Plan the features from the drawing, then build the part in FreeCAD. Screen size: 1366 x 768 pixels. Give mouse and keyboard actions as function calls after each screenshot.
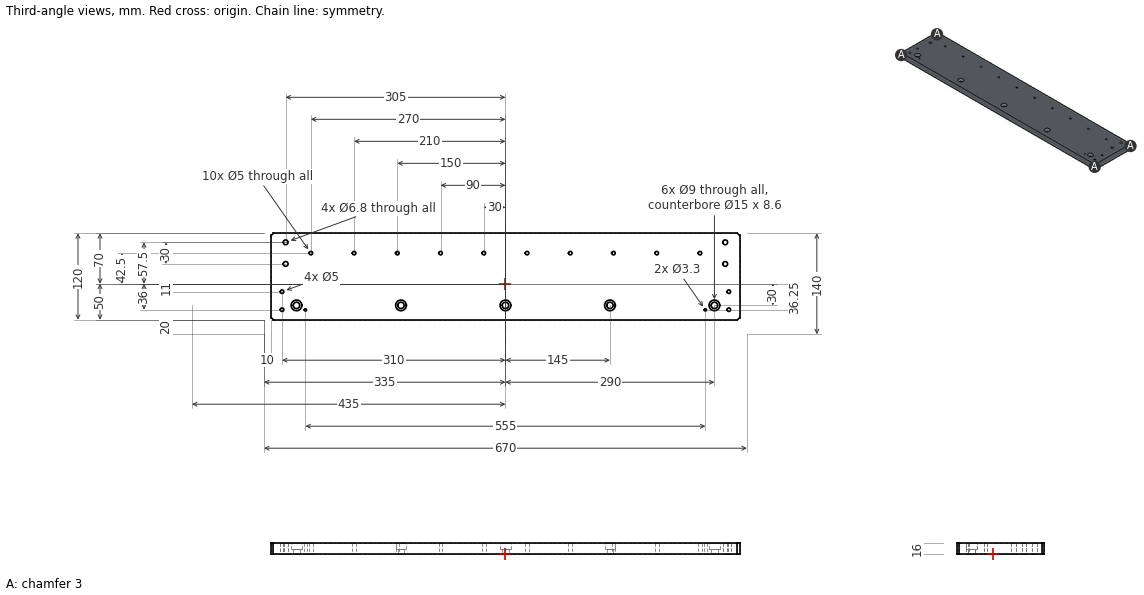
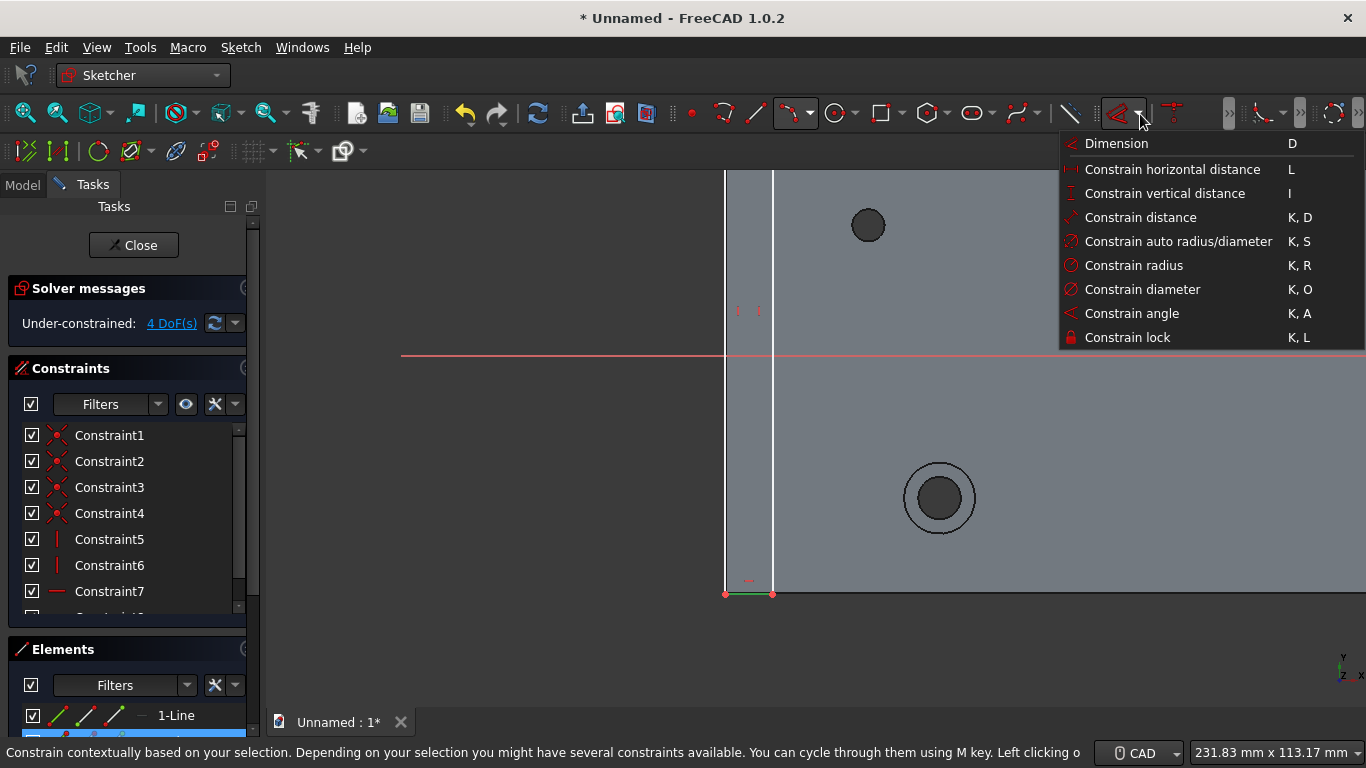
click(1212, 169)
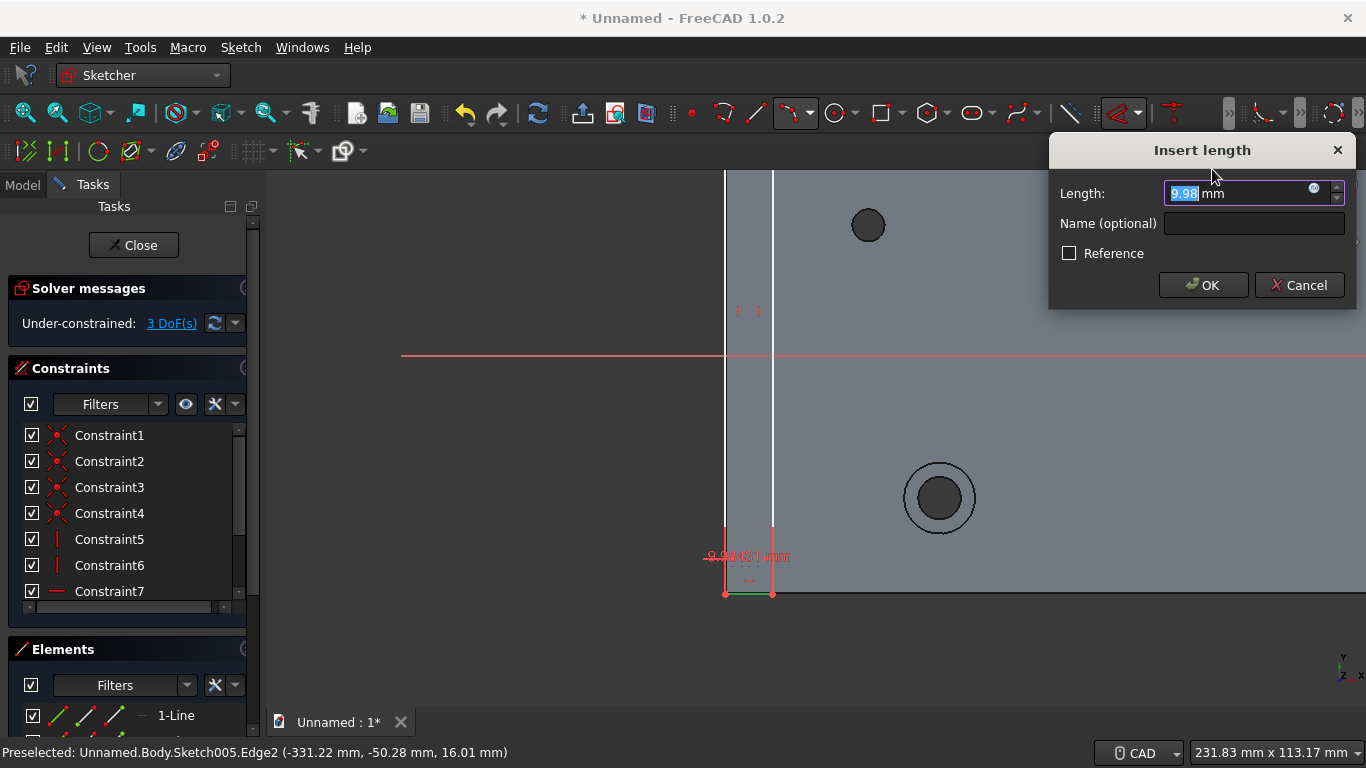
text(10)
key(Return)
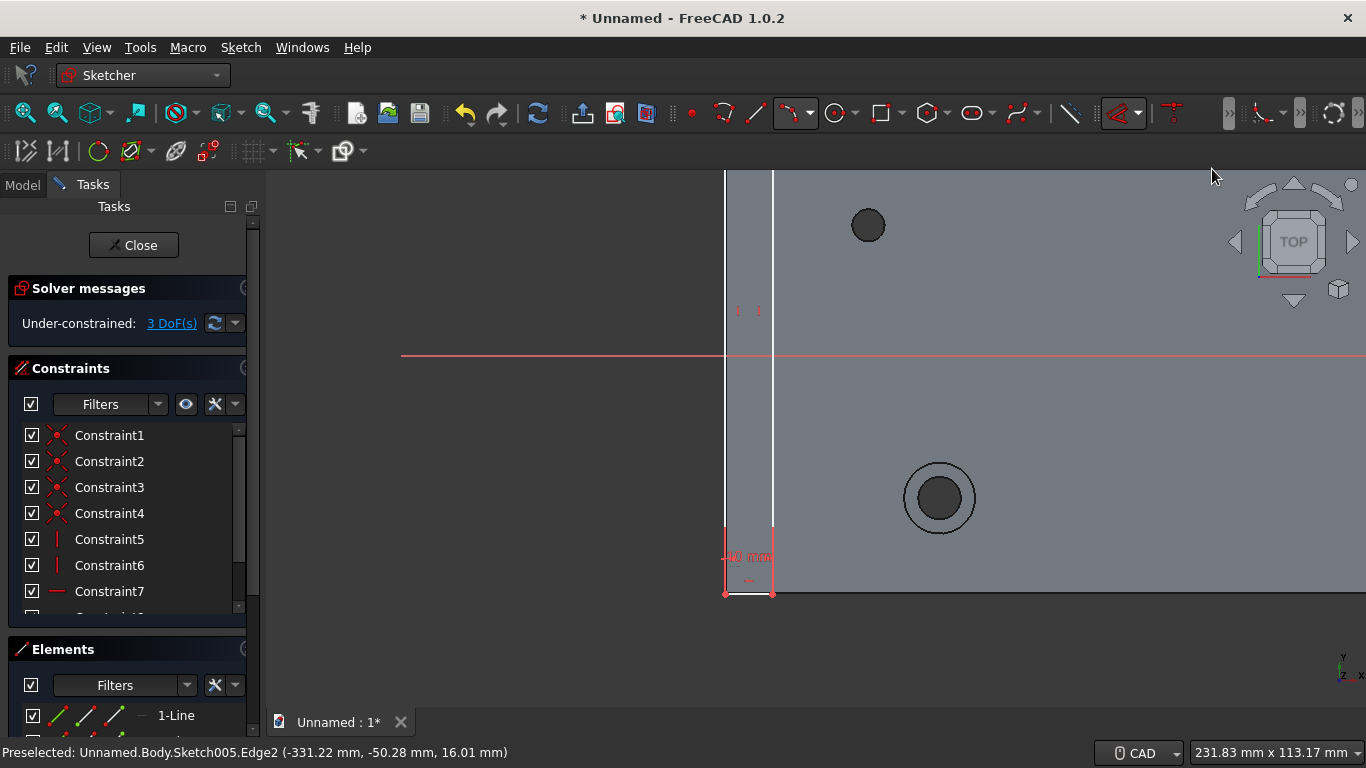
click(725, 424)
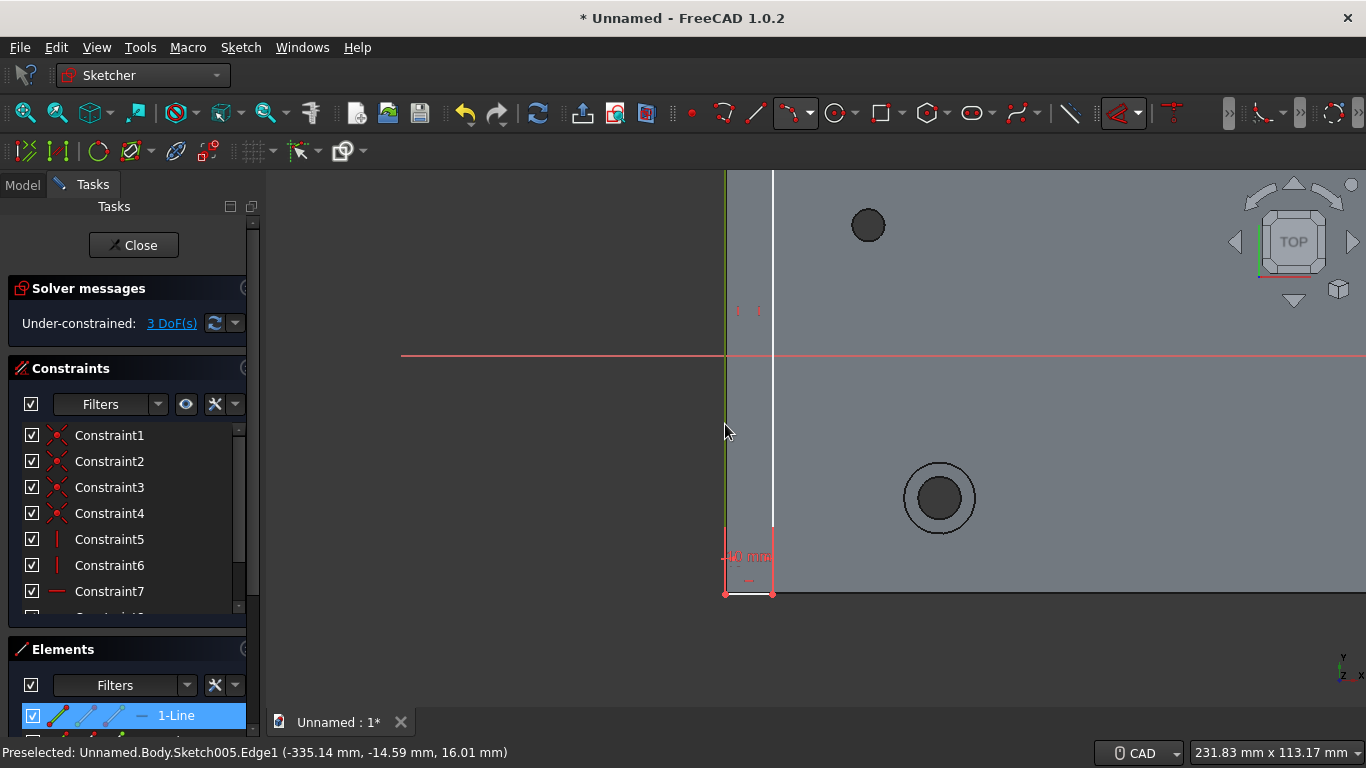
click(1140, 114)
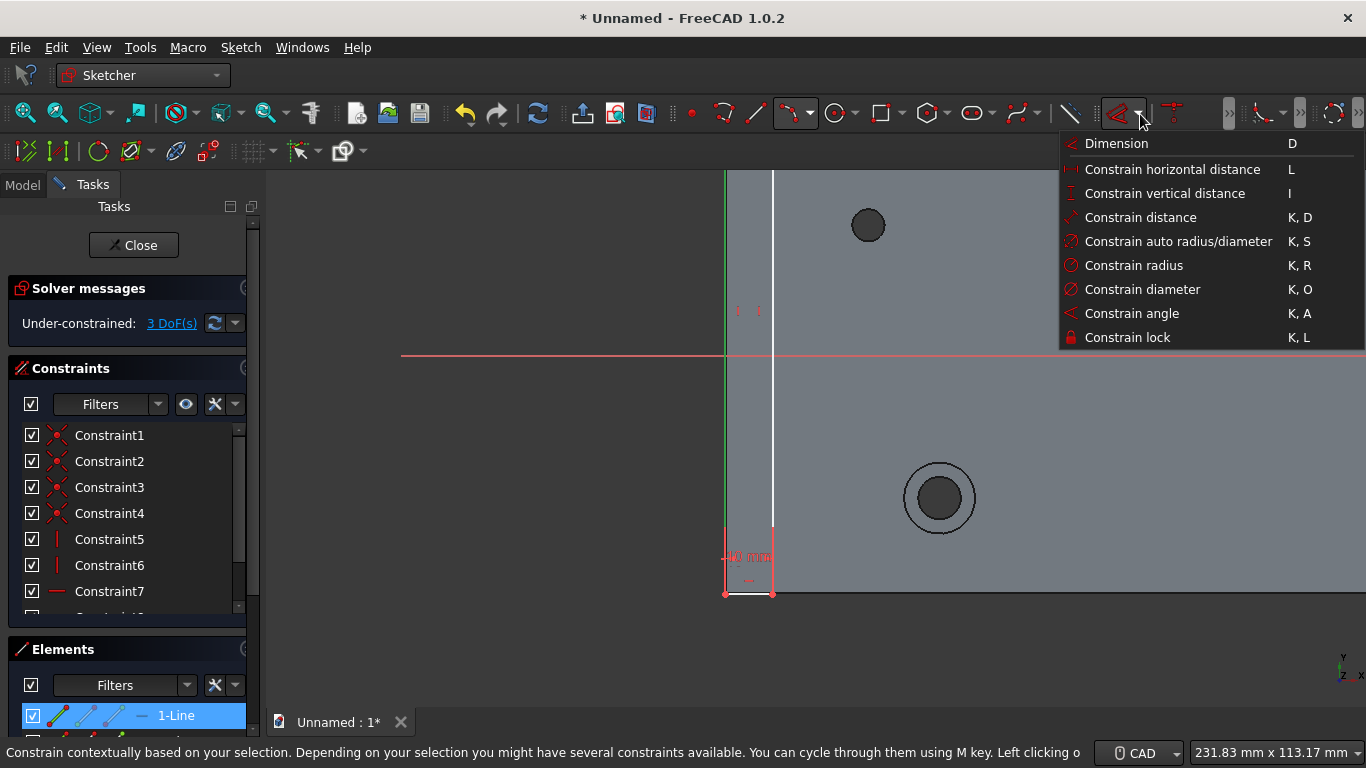
click(1212, 193)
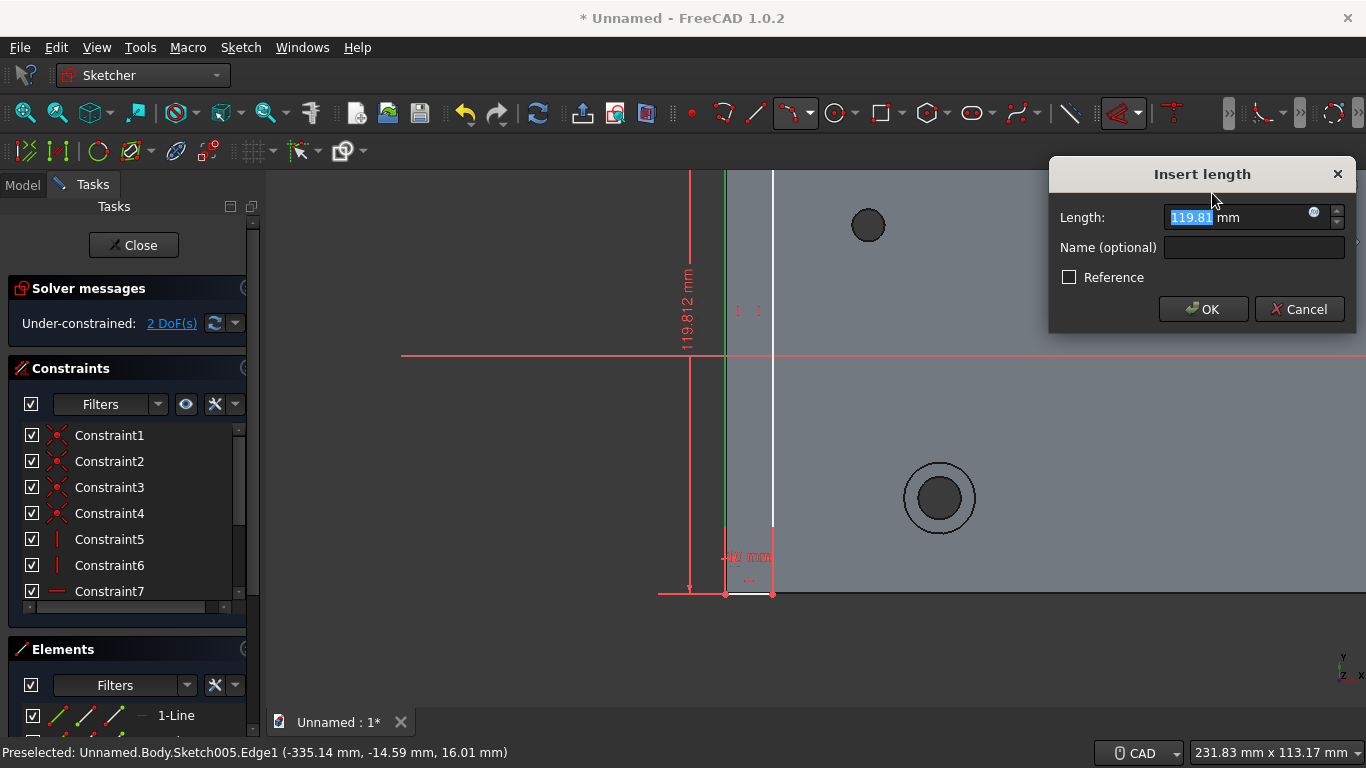
text(120)
key(Return)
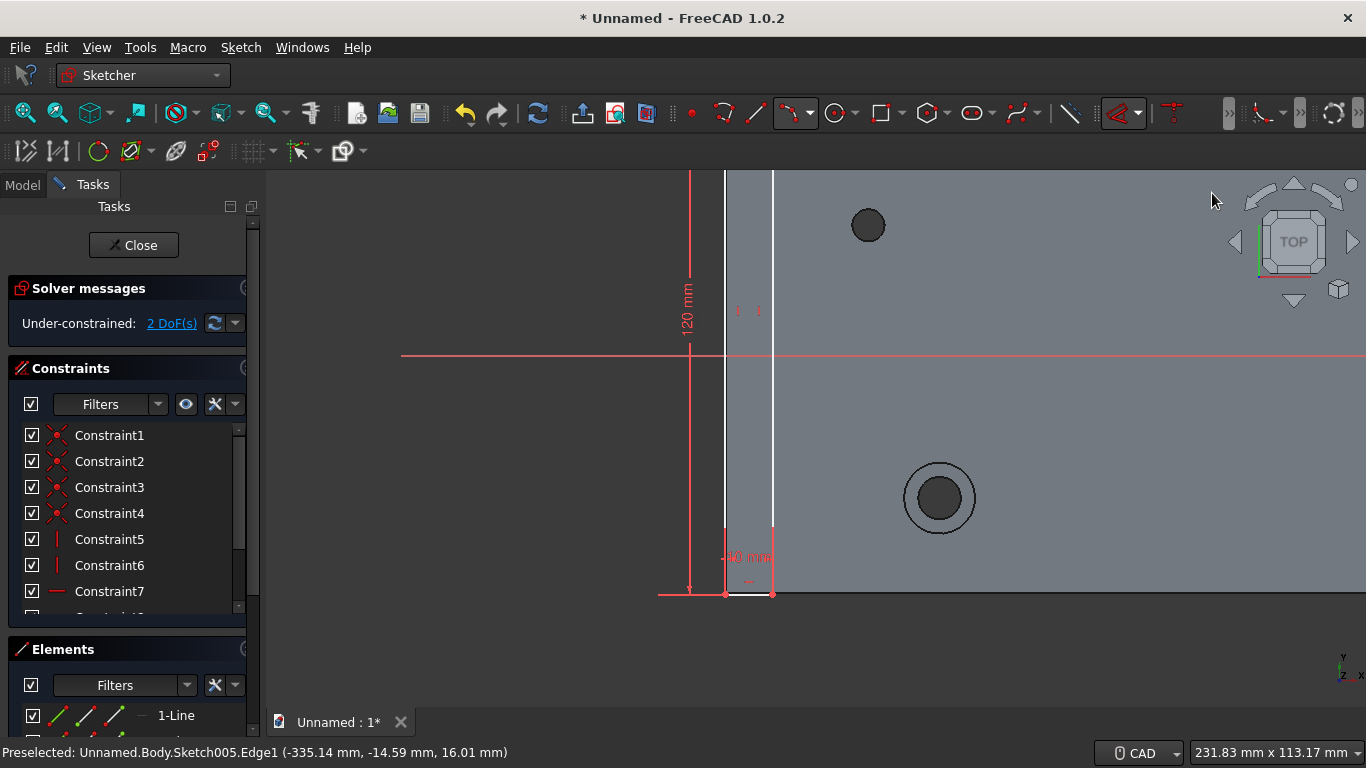
scroll(745, 597, down, 3)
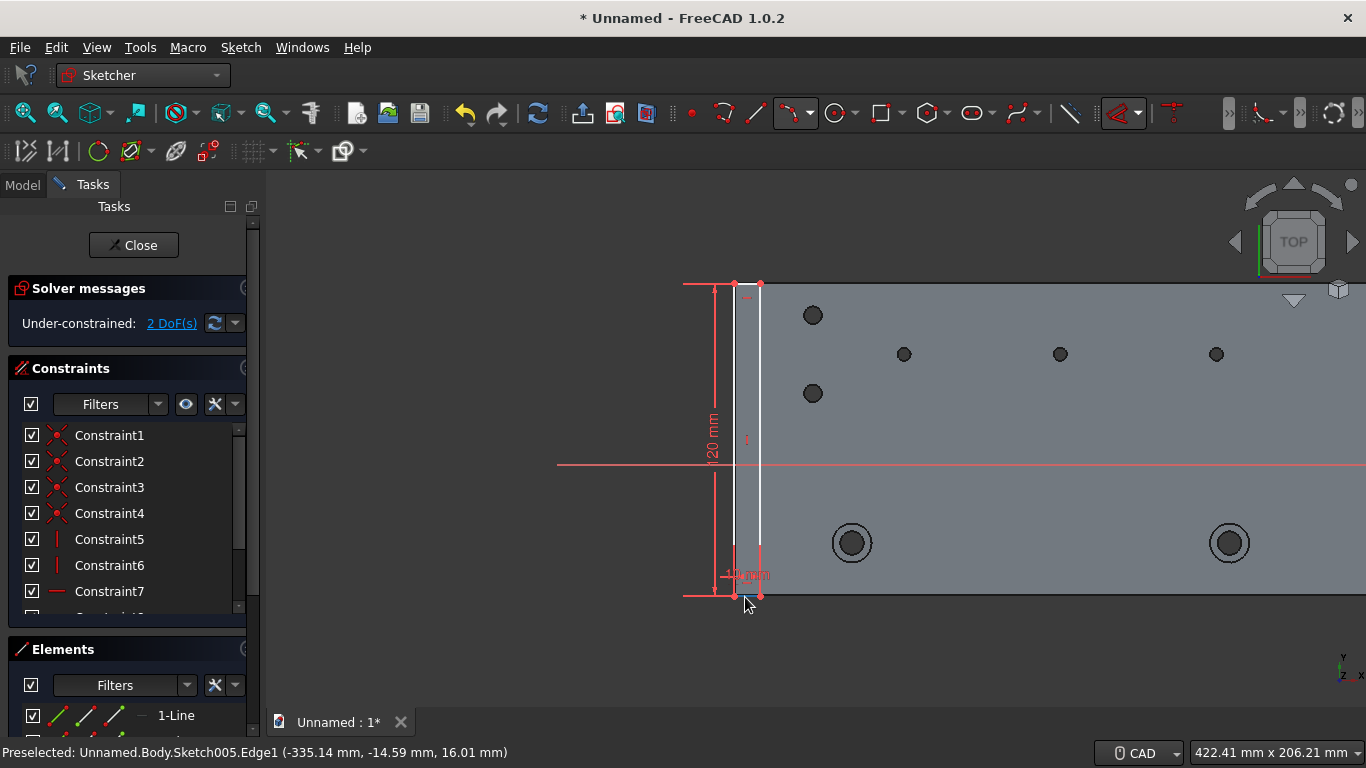
click(734, 284)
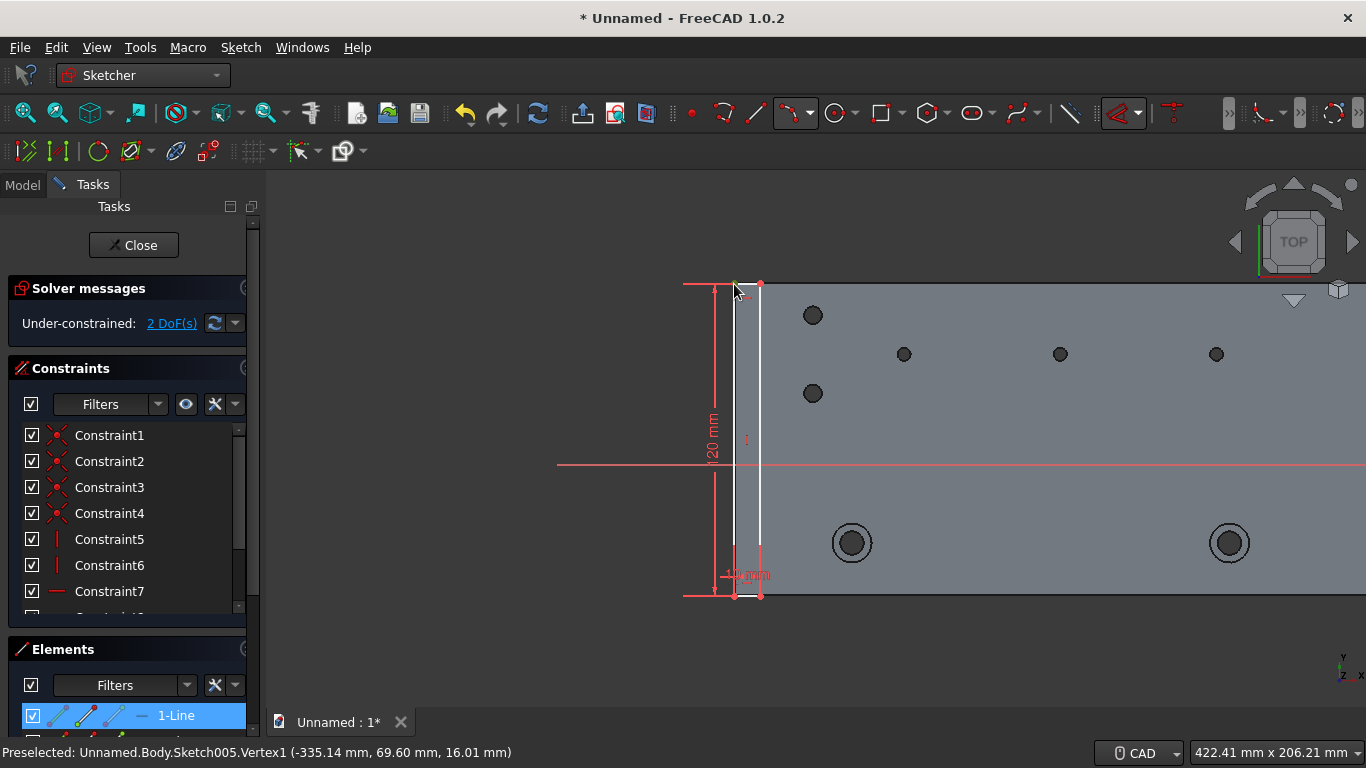
key(i)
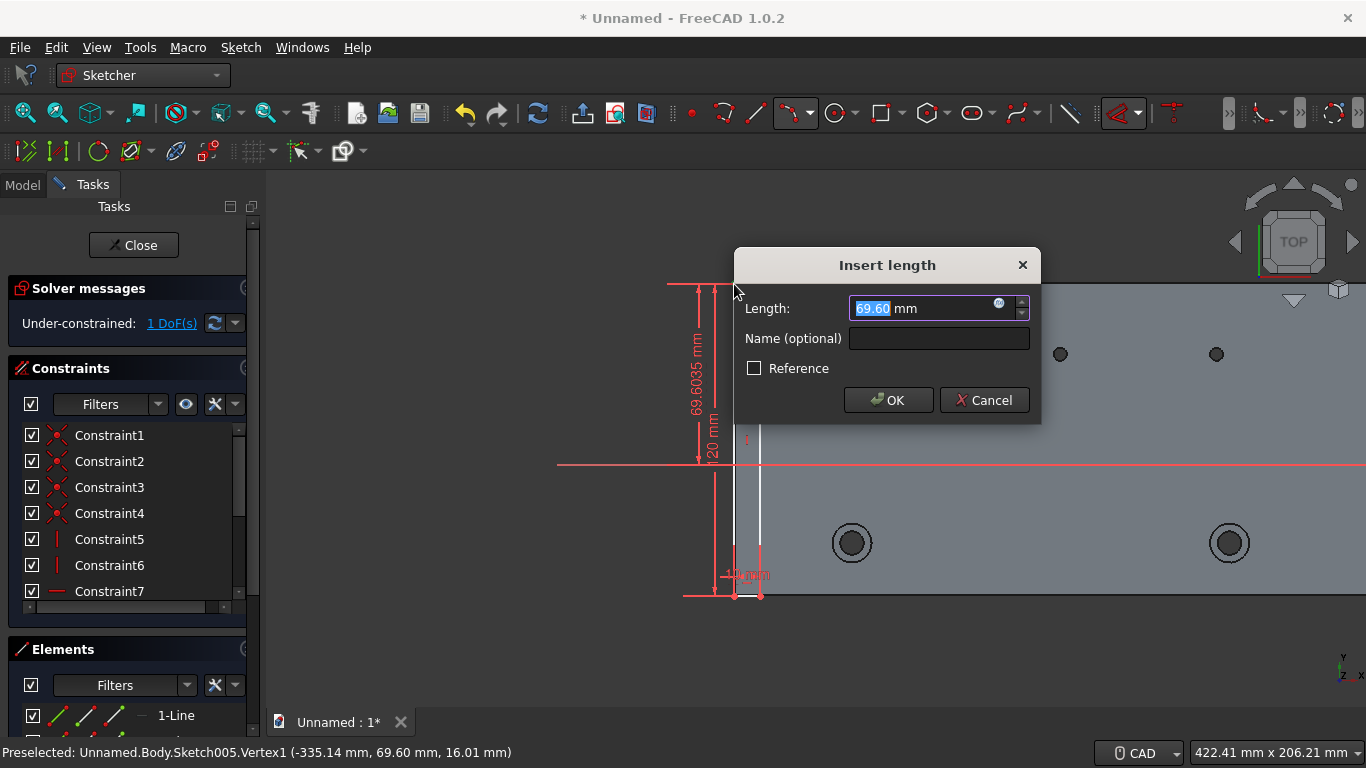
text(70)
key(Return)